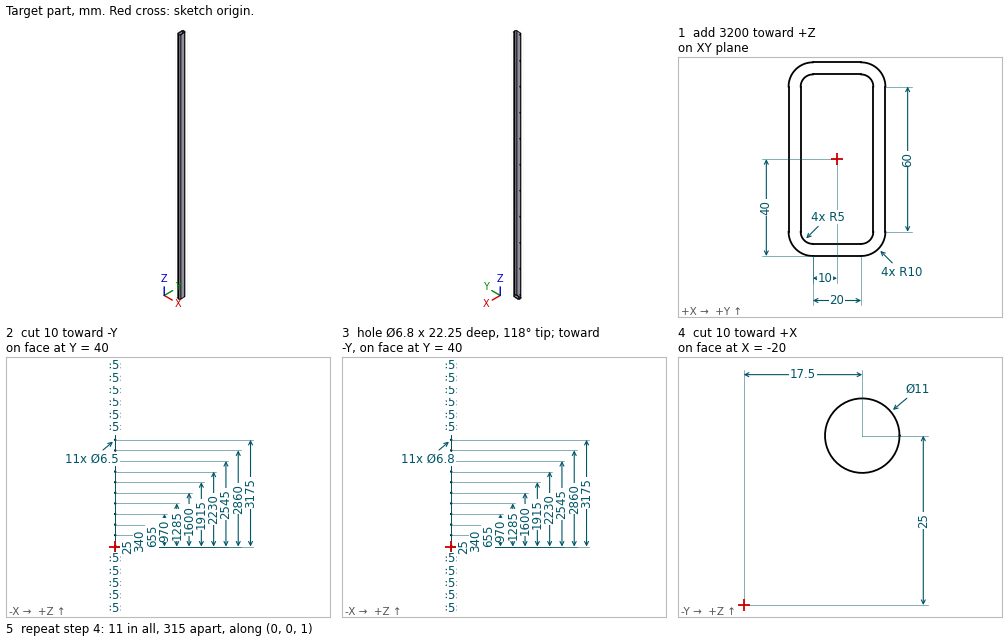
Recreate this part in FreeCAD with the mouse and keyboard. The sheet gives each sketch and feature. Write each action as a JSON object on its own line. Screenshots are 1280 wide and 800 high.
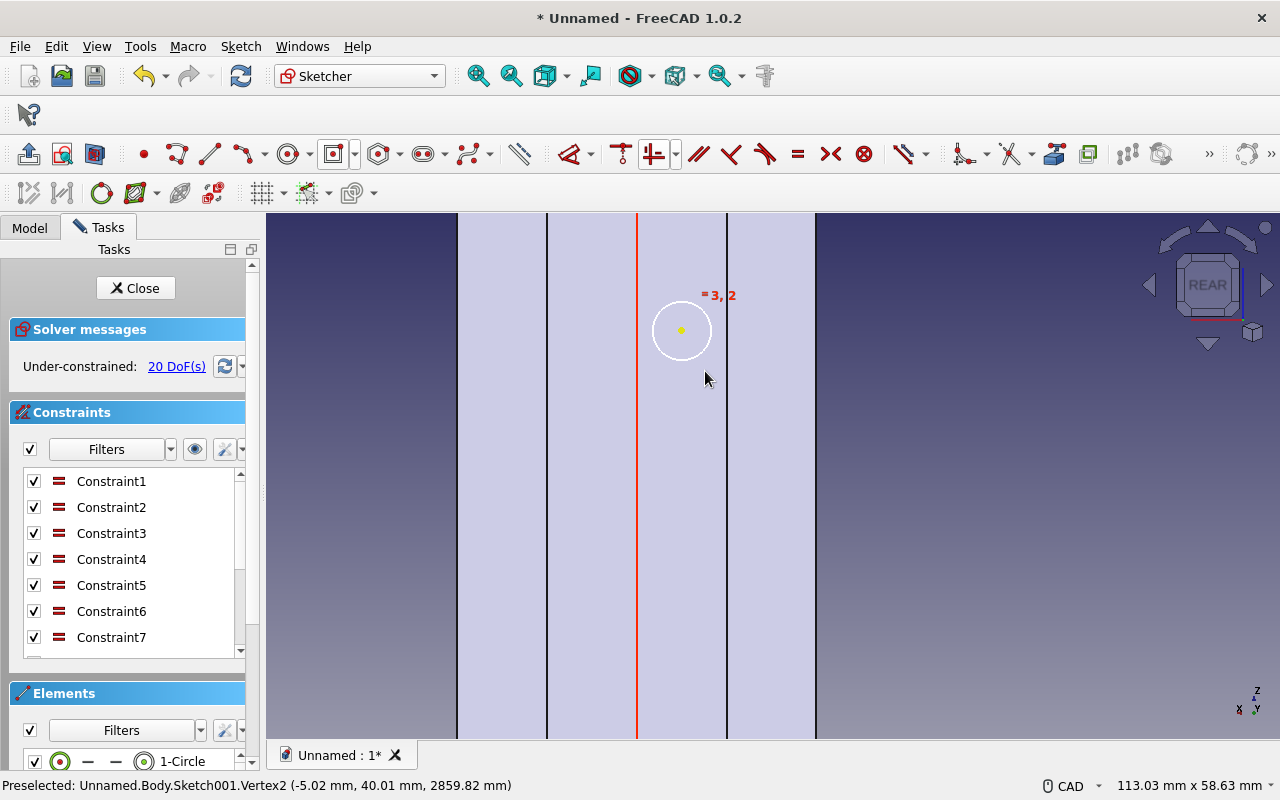
{"action": "left_click", "coordinate": [682, 331]}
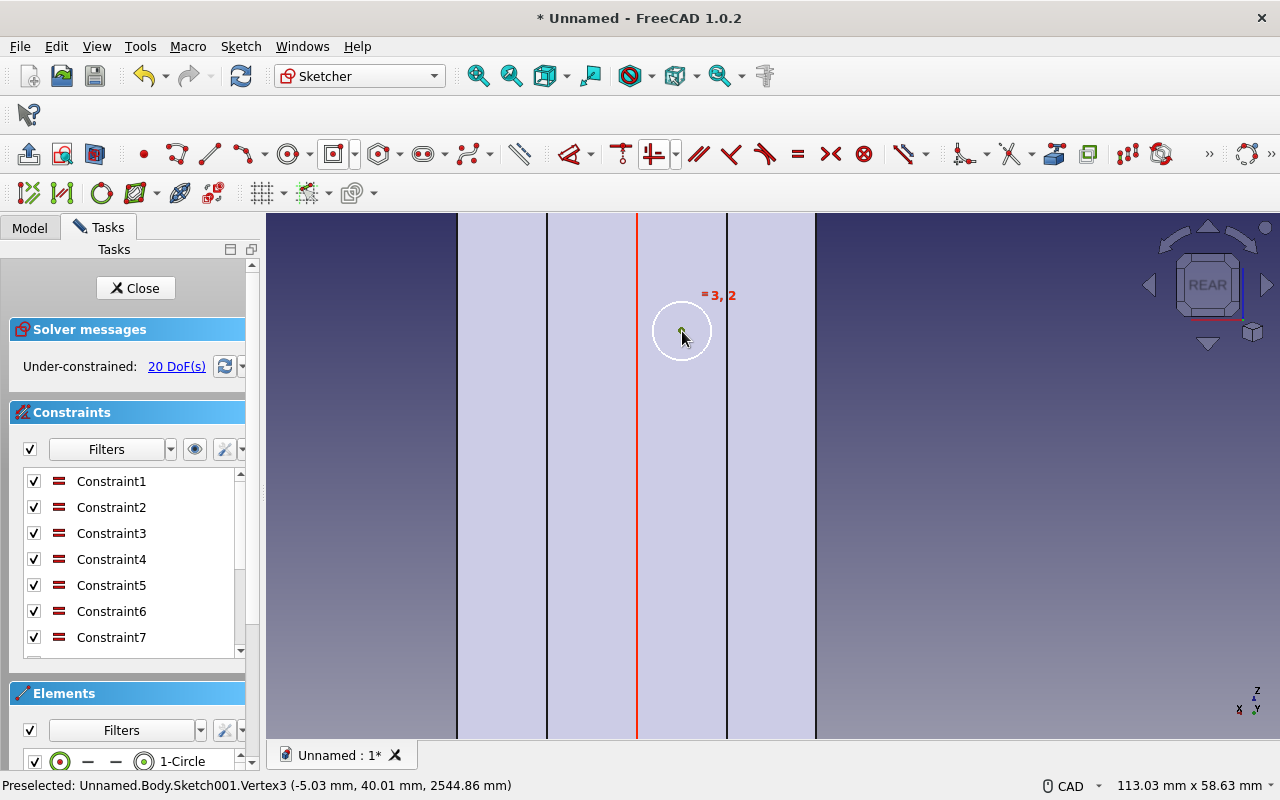
{"action": "key", "text": "l"}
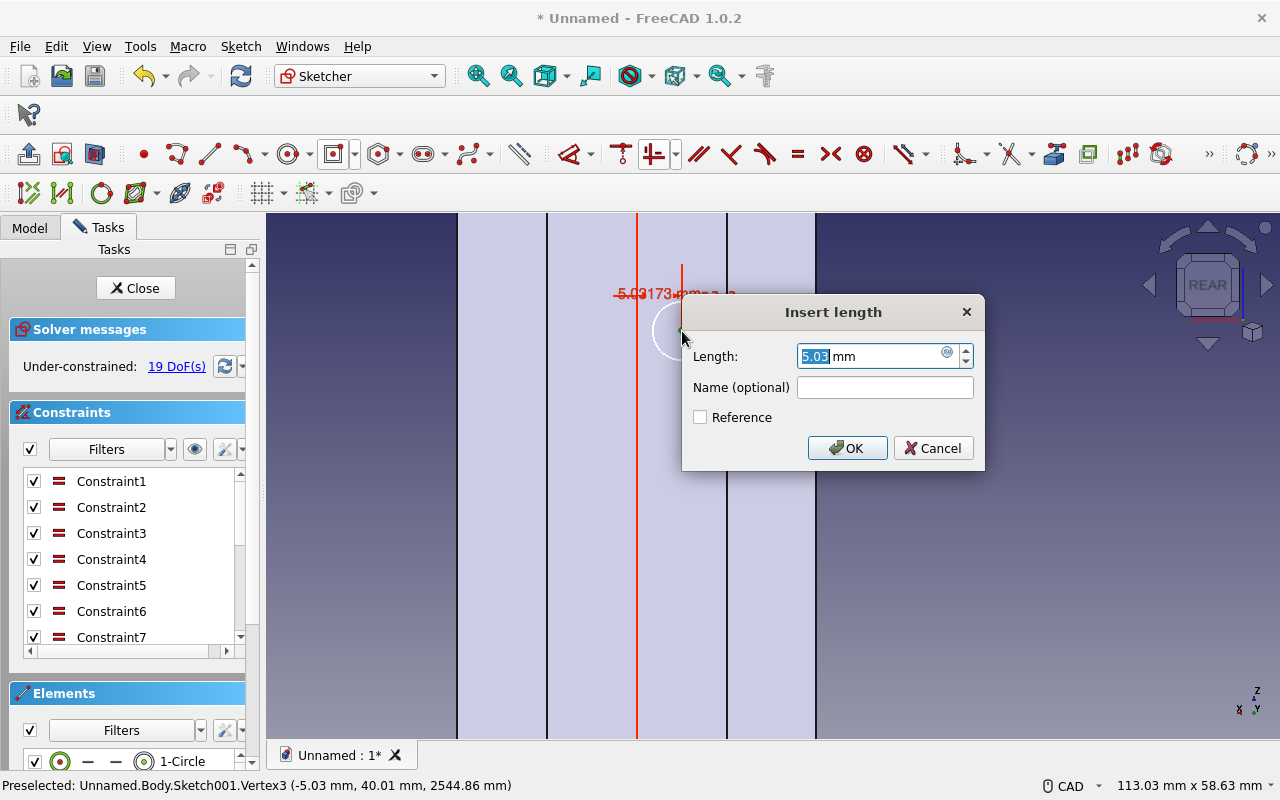
{"action": "type", "text": "5"}
{"action": "key", "text": "Return"}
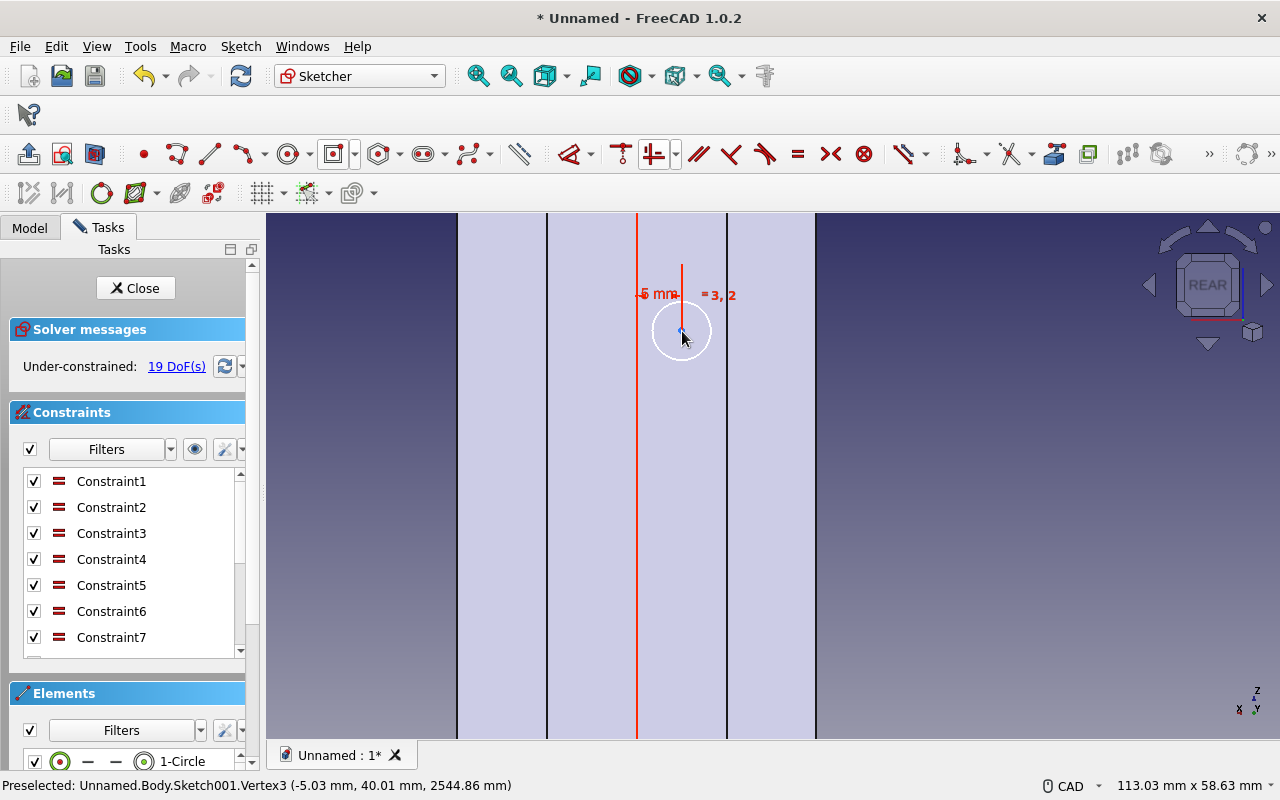
{"action": "scroll", "coordinate": [704, 476], "scroll_direction": "down", "scroll_amount": 15}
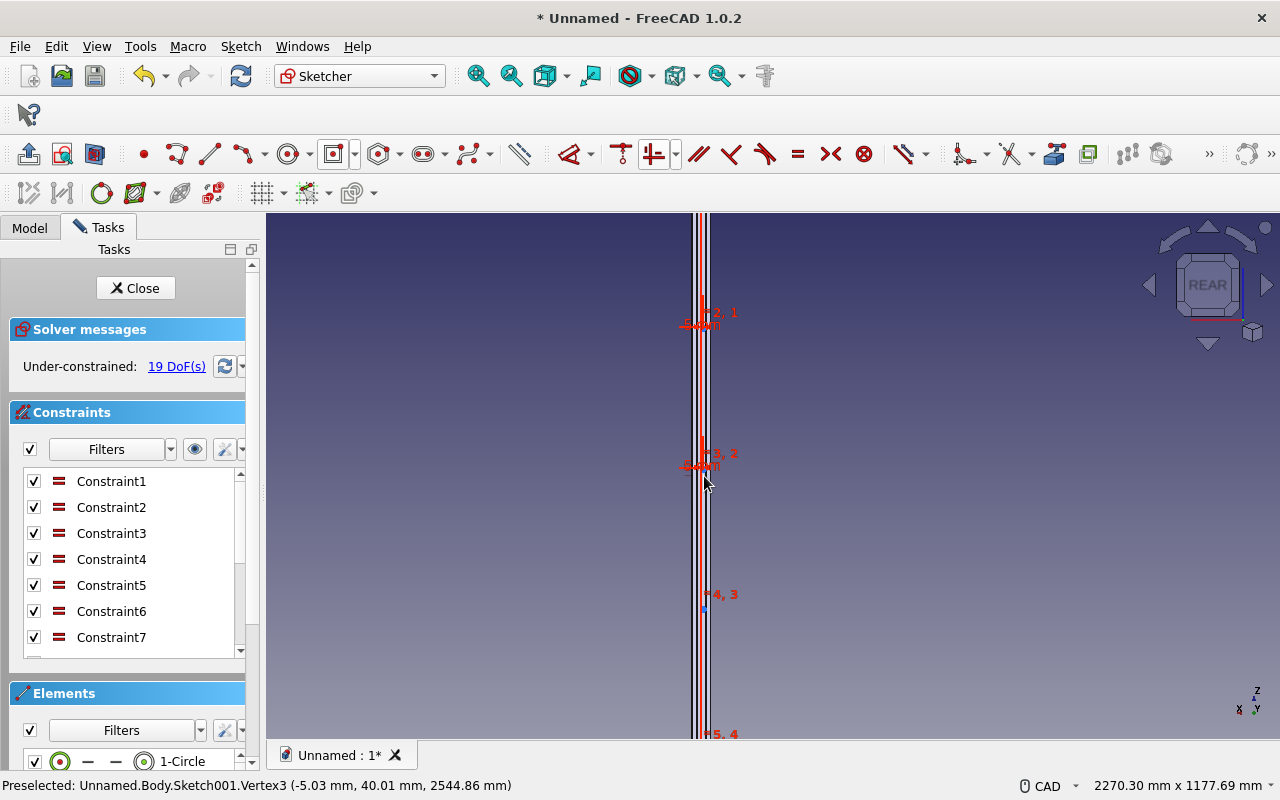
{"action": "scroll", "coordinate": [705, 338], "scroll_direction": "down", "scroll_amount": 7}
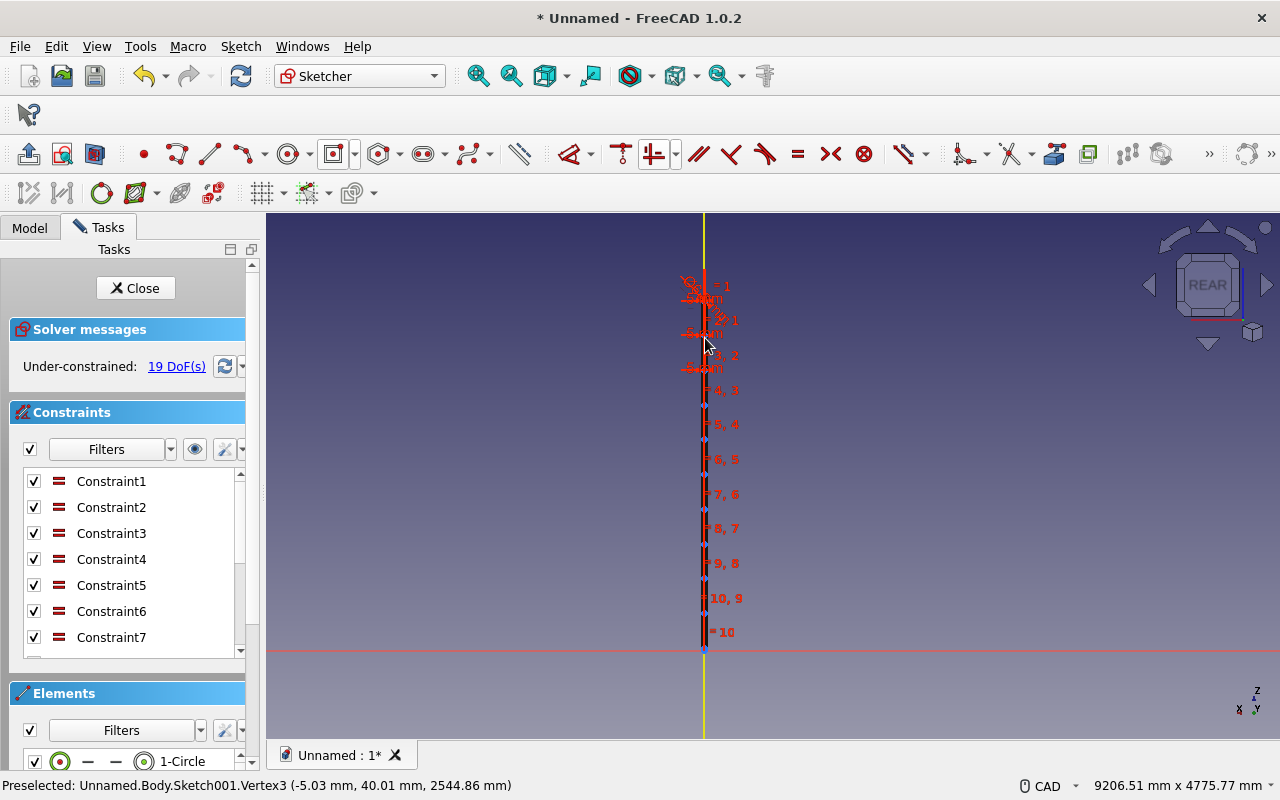
{"action": "scroll", "coordinate": [705, 405], "scroll_direction": "up", "scroll_amount": 22}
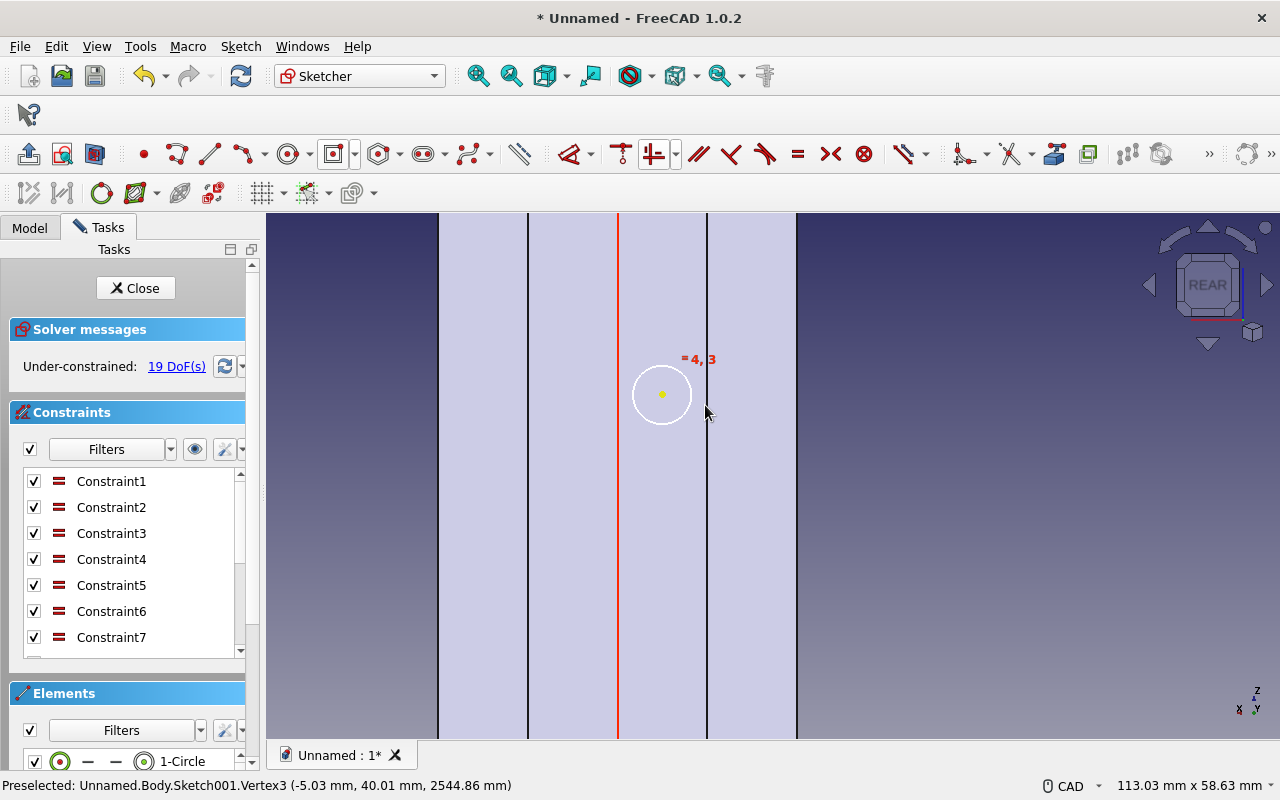
{"action": "left_click", "coordinate": [662, 395]}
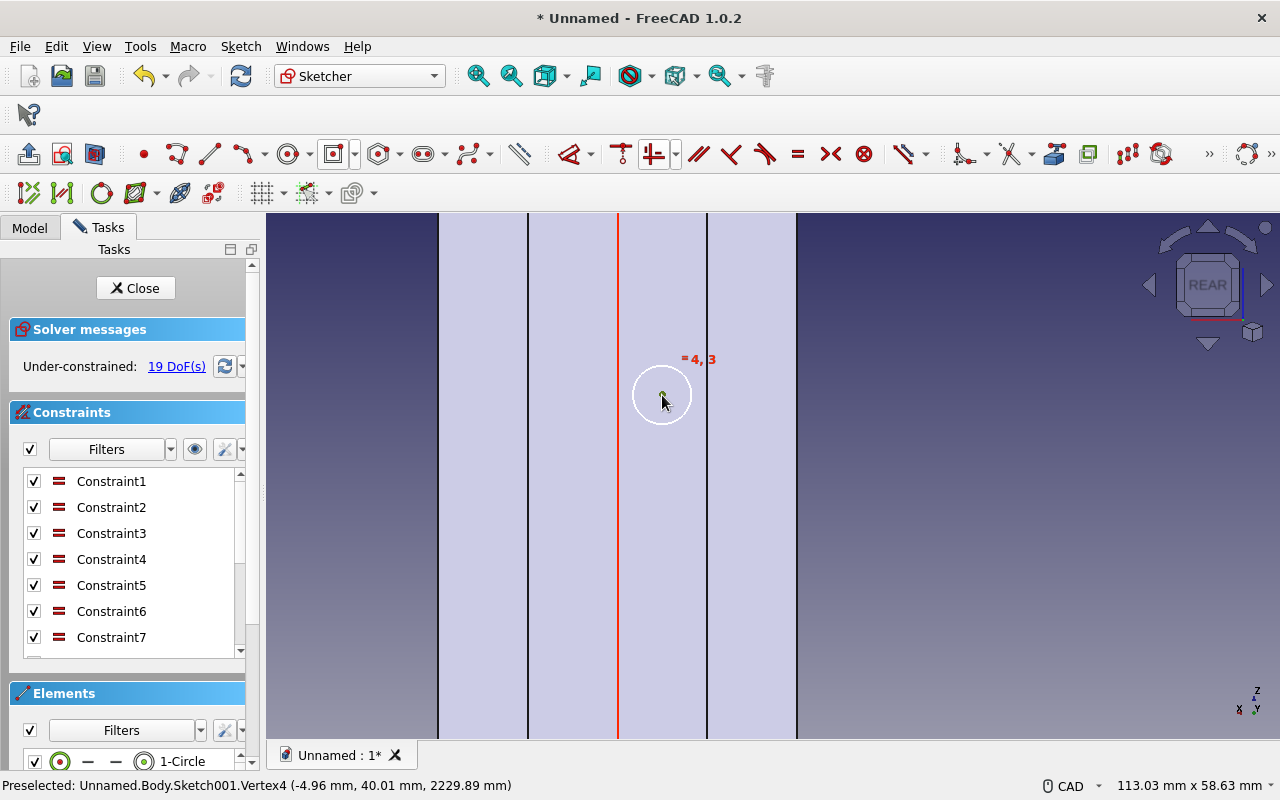
{"action": "key", "text": "l"}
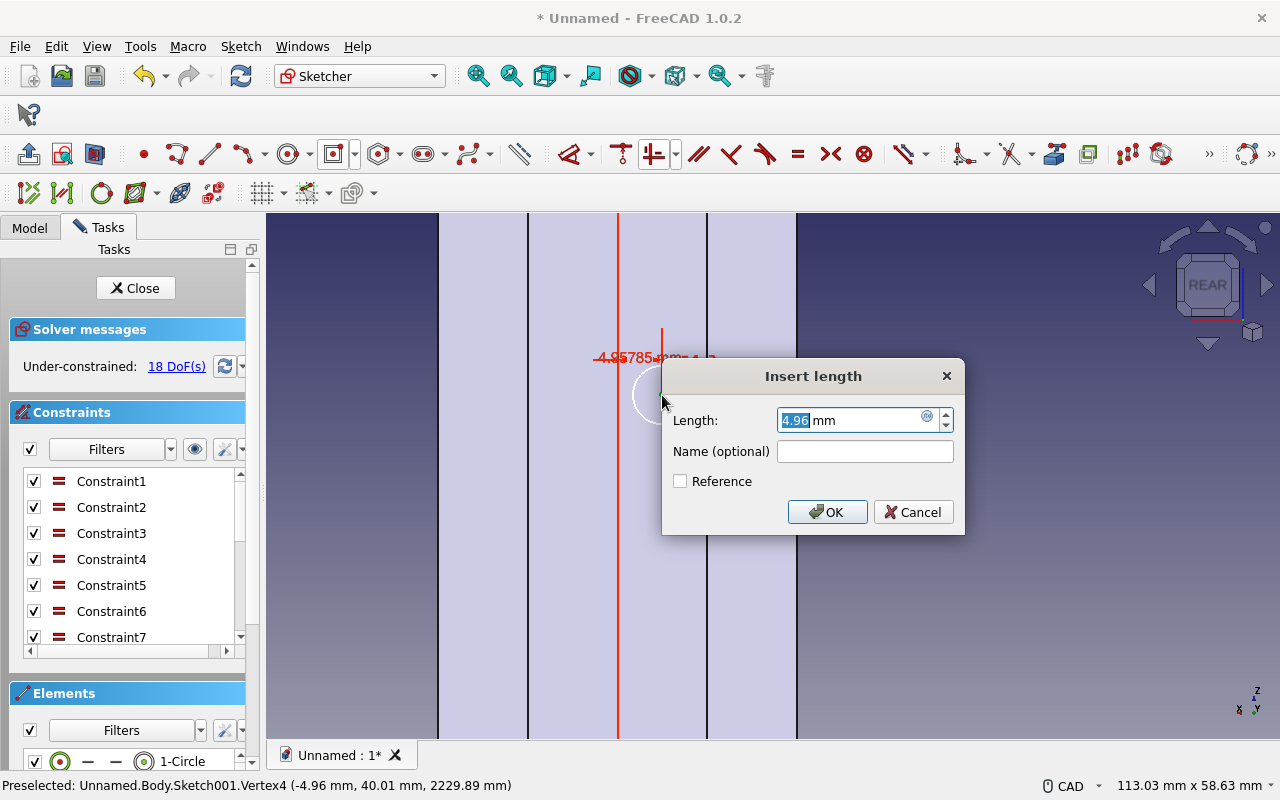
{"action": "type", "text": "5"}
{"action": "key", "text": "Return"}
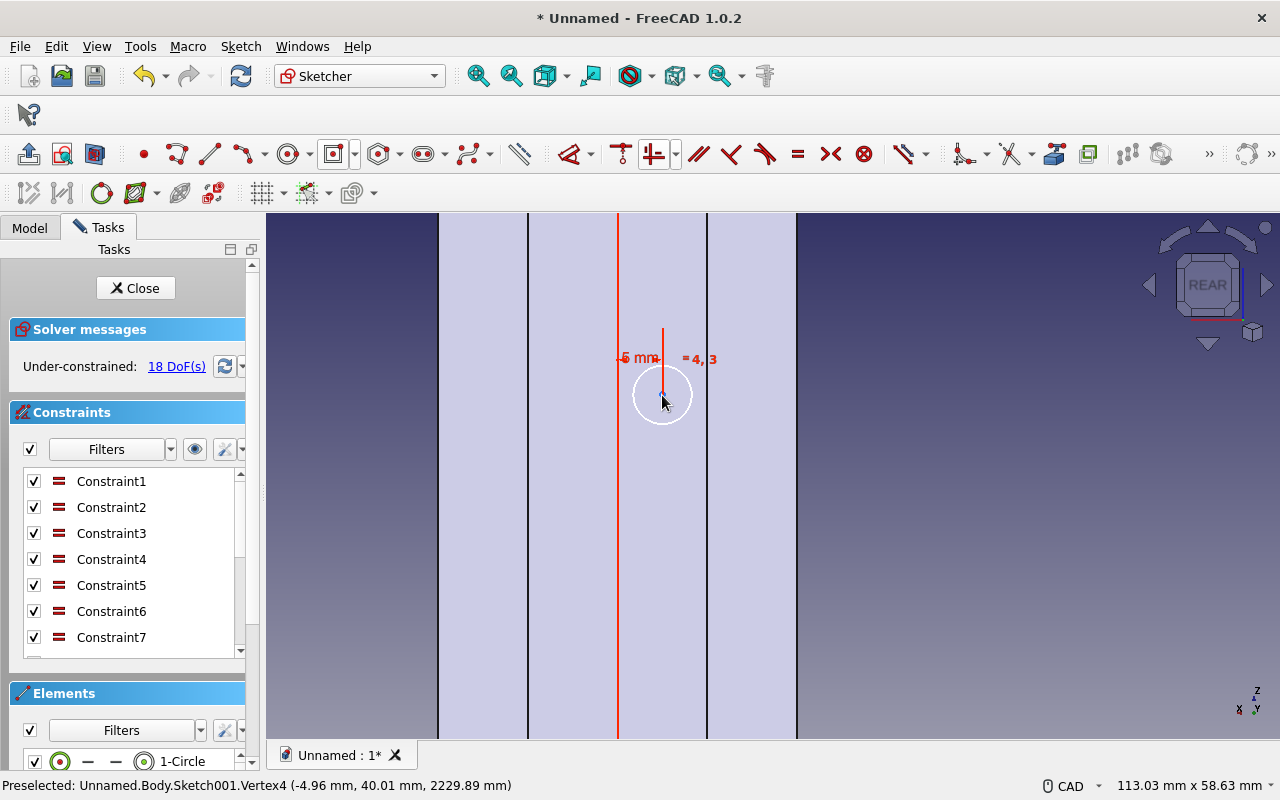
{"action": "scroll", "coordinate": [704, 476], "scroll_direction": "down", "scroll_amount": 15}